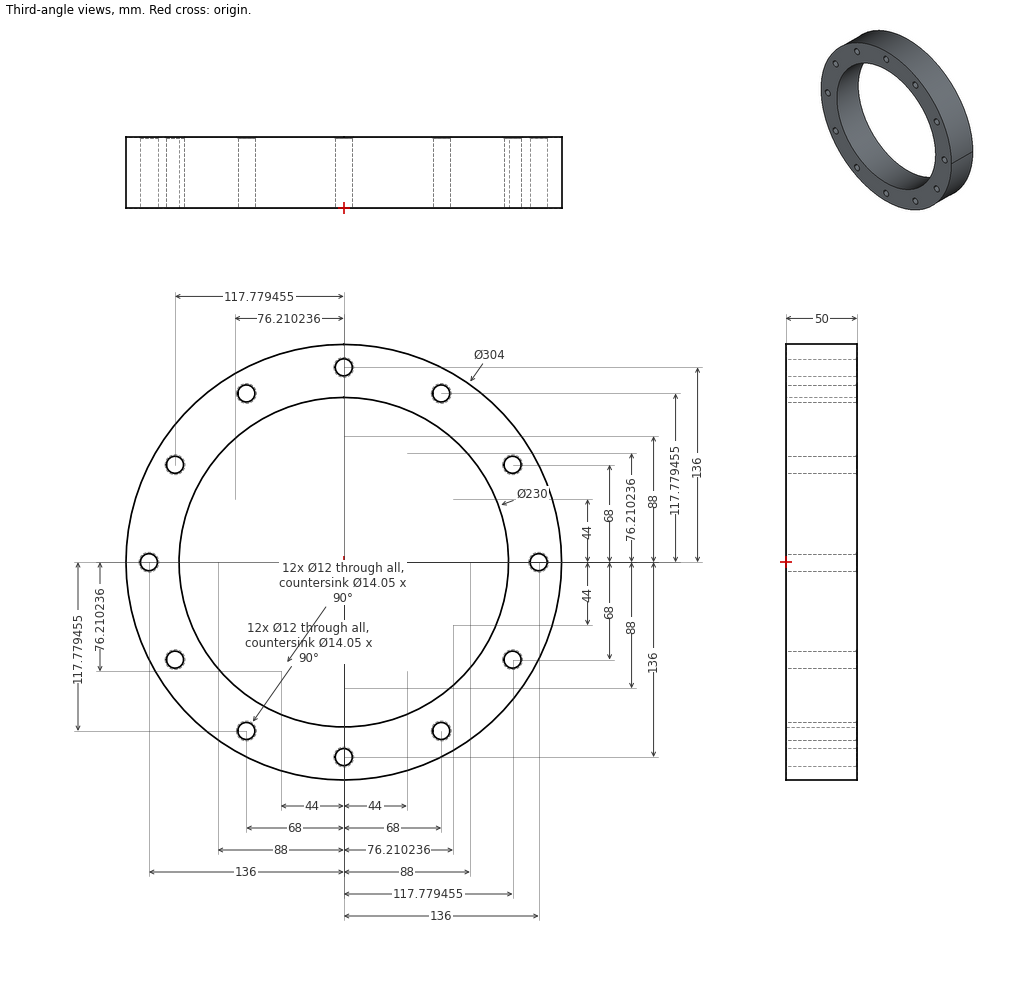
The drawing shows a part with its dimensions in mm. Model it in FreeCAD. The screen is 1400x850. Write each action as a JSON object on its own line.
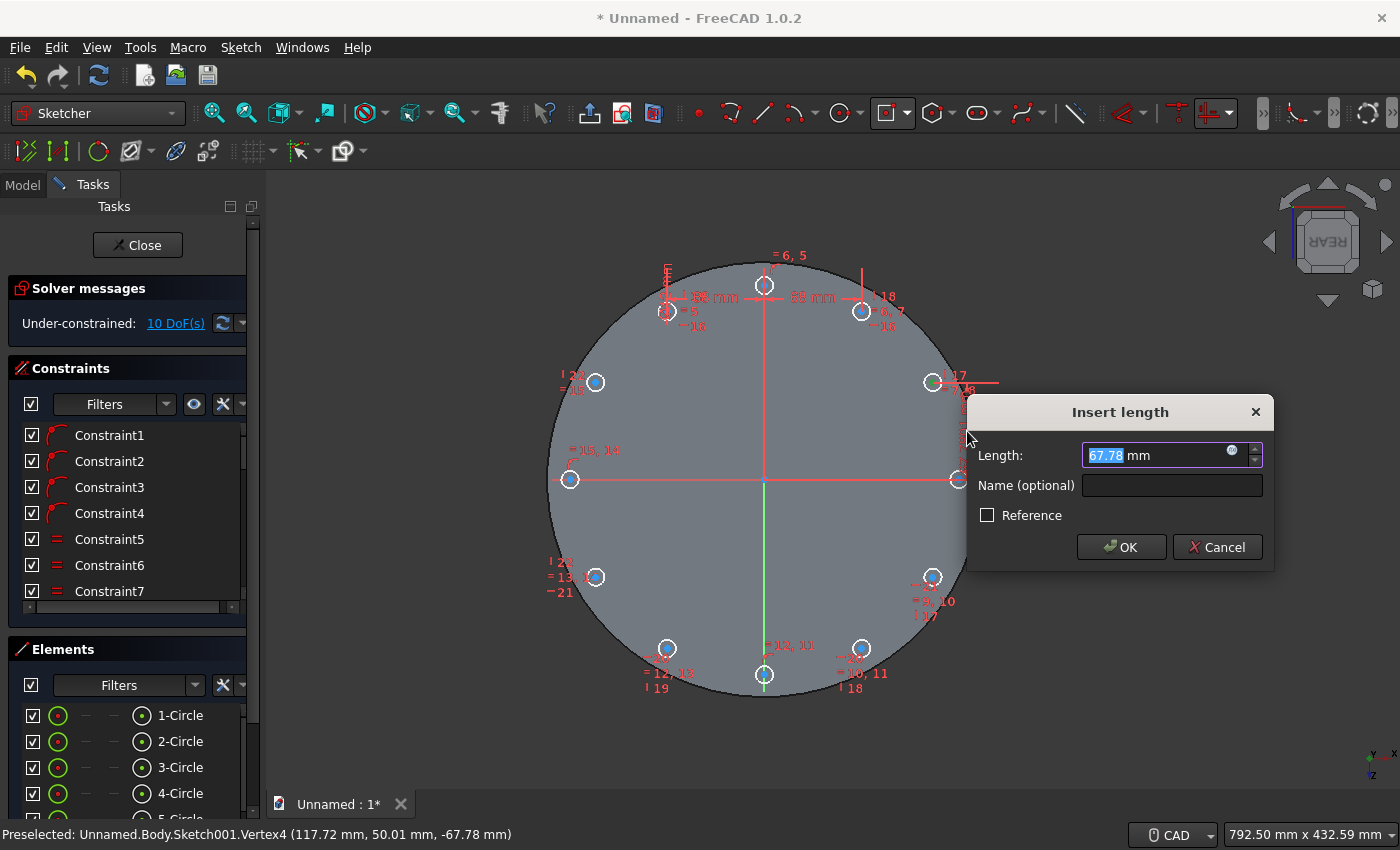
{"action": "type", "text": "68"}
{"action": "key", "text": "Return"}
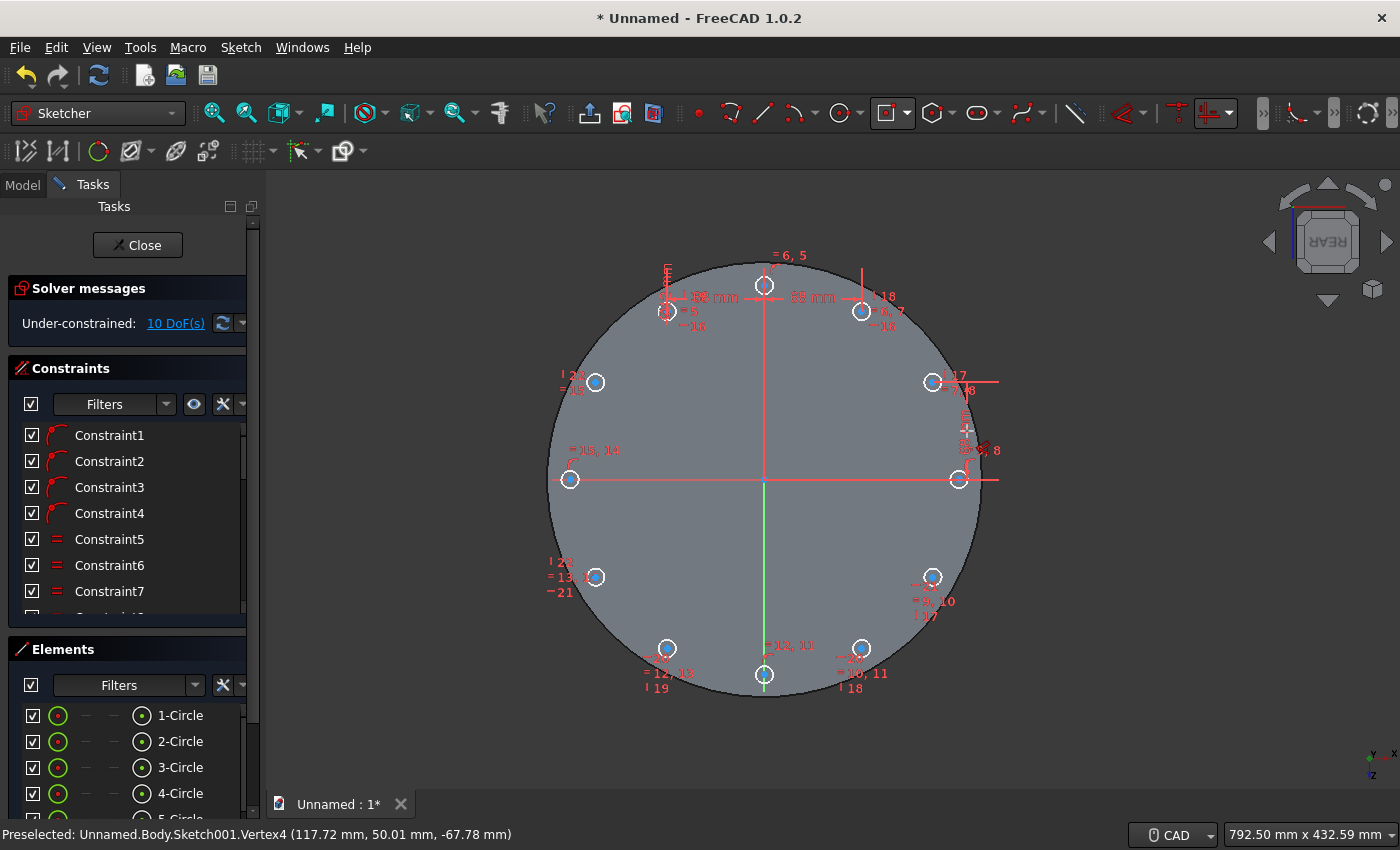
{"action": "left_click", "coordinate": [933, 577]}
{"action": "left_click", "coordinate": [967, 528]}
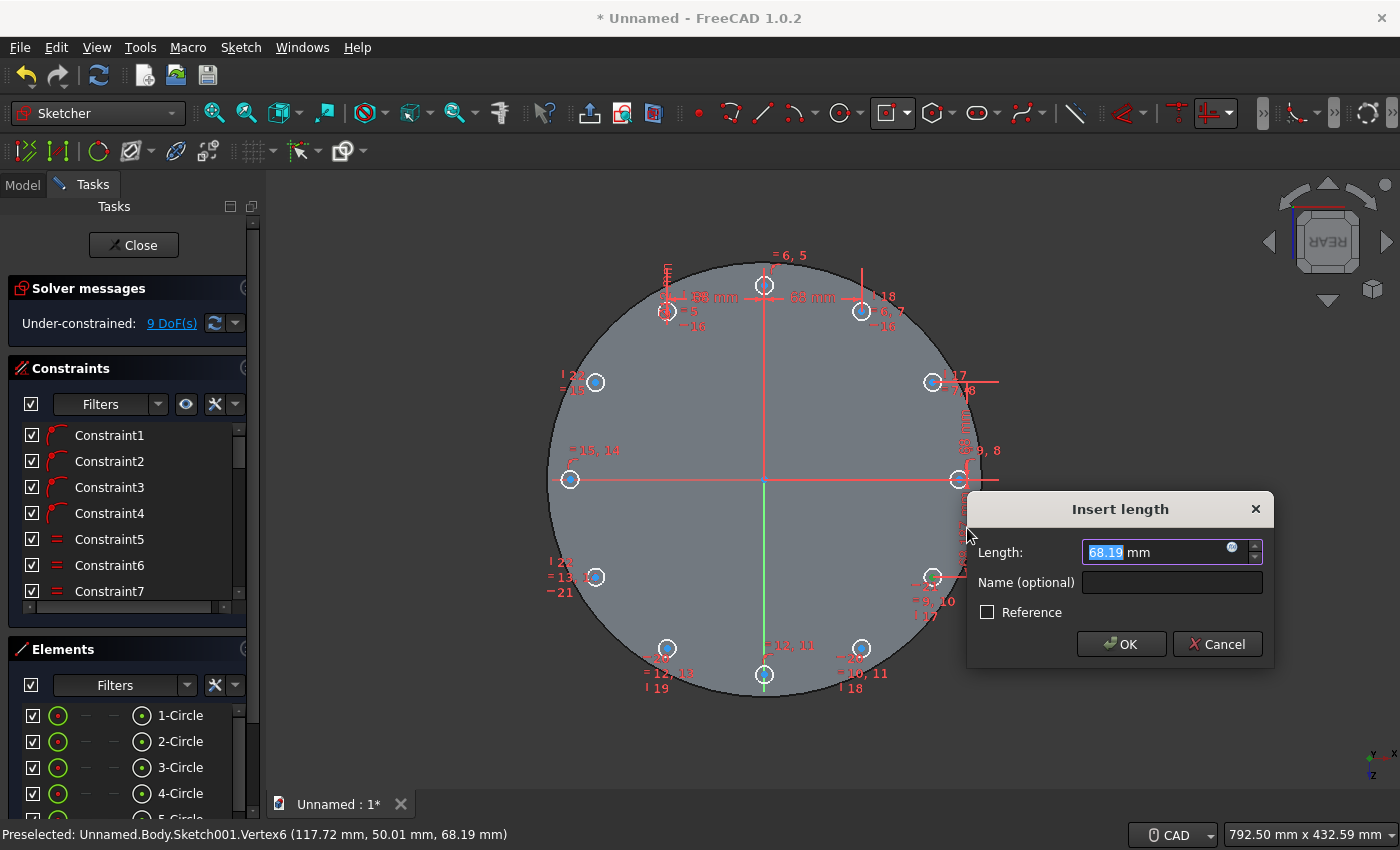
{"action": "type", "text": "68"}
{"action": "key", "text": "Return"}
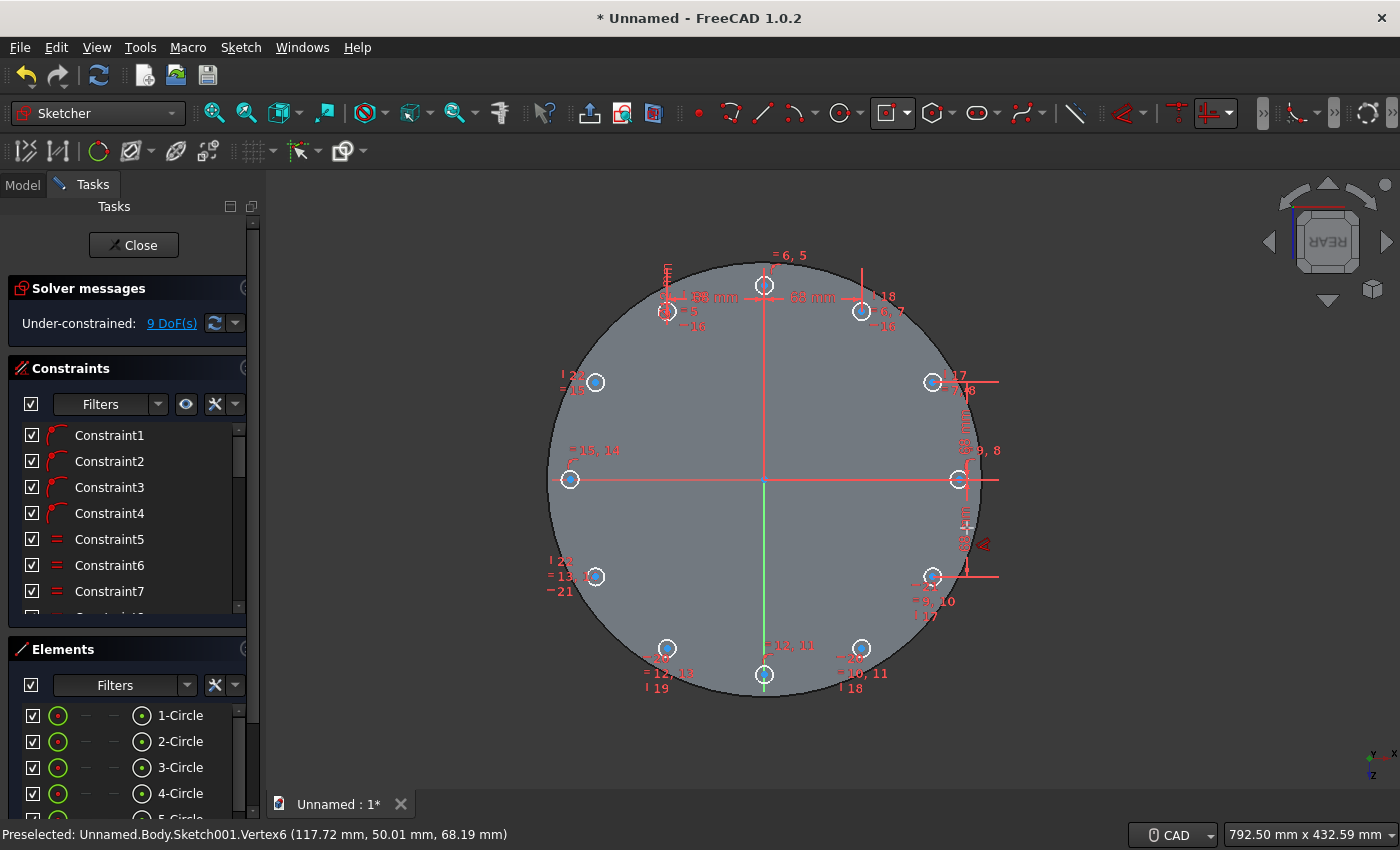
{"action": "left_click", "coordinate": [596, 383]}
{"action": "left_click", "coordinate": [562, 431]}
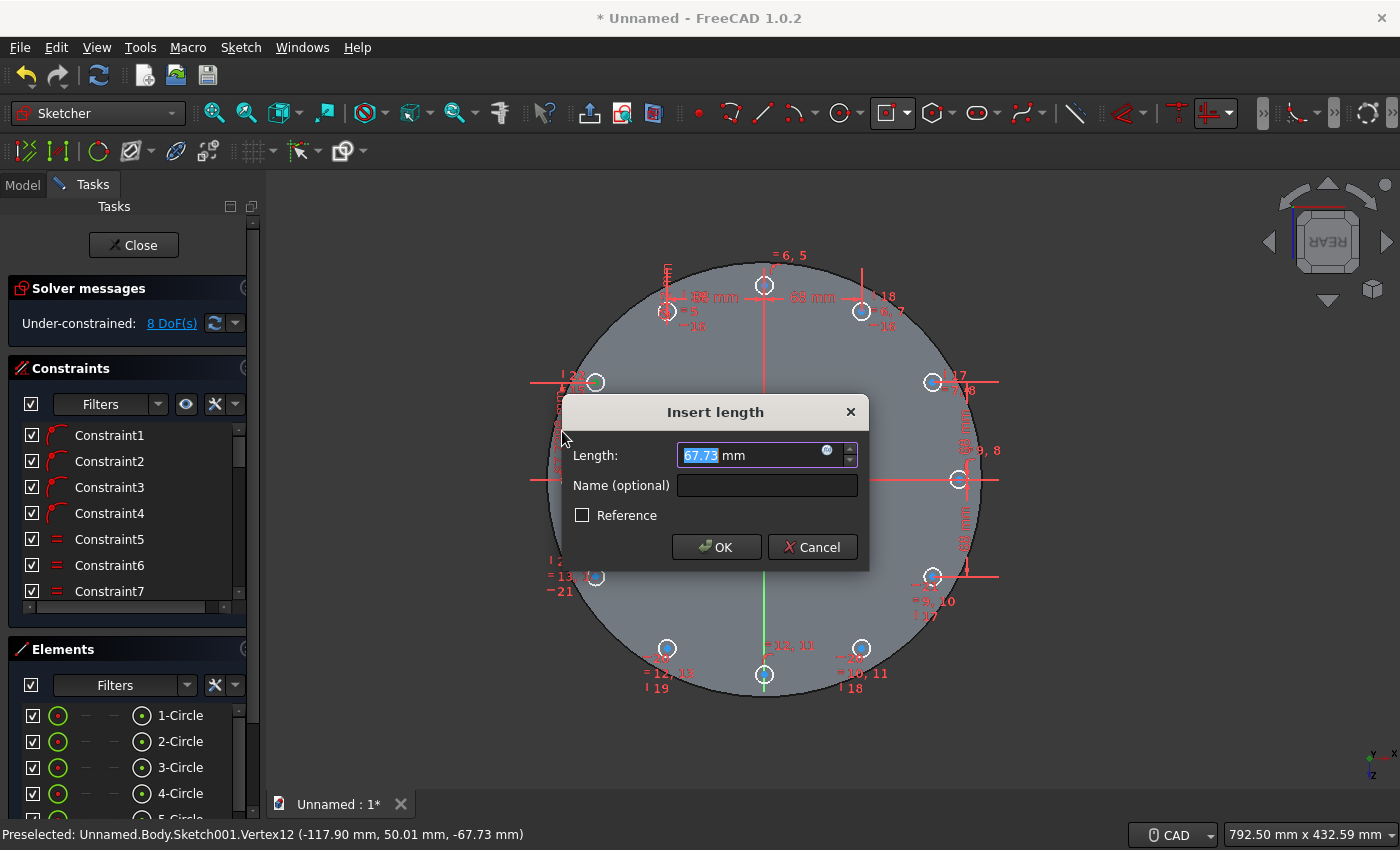
{"action": "type", "text": "68"}
{"action": "key", "text": "Return"}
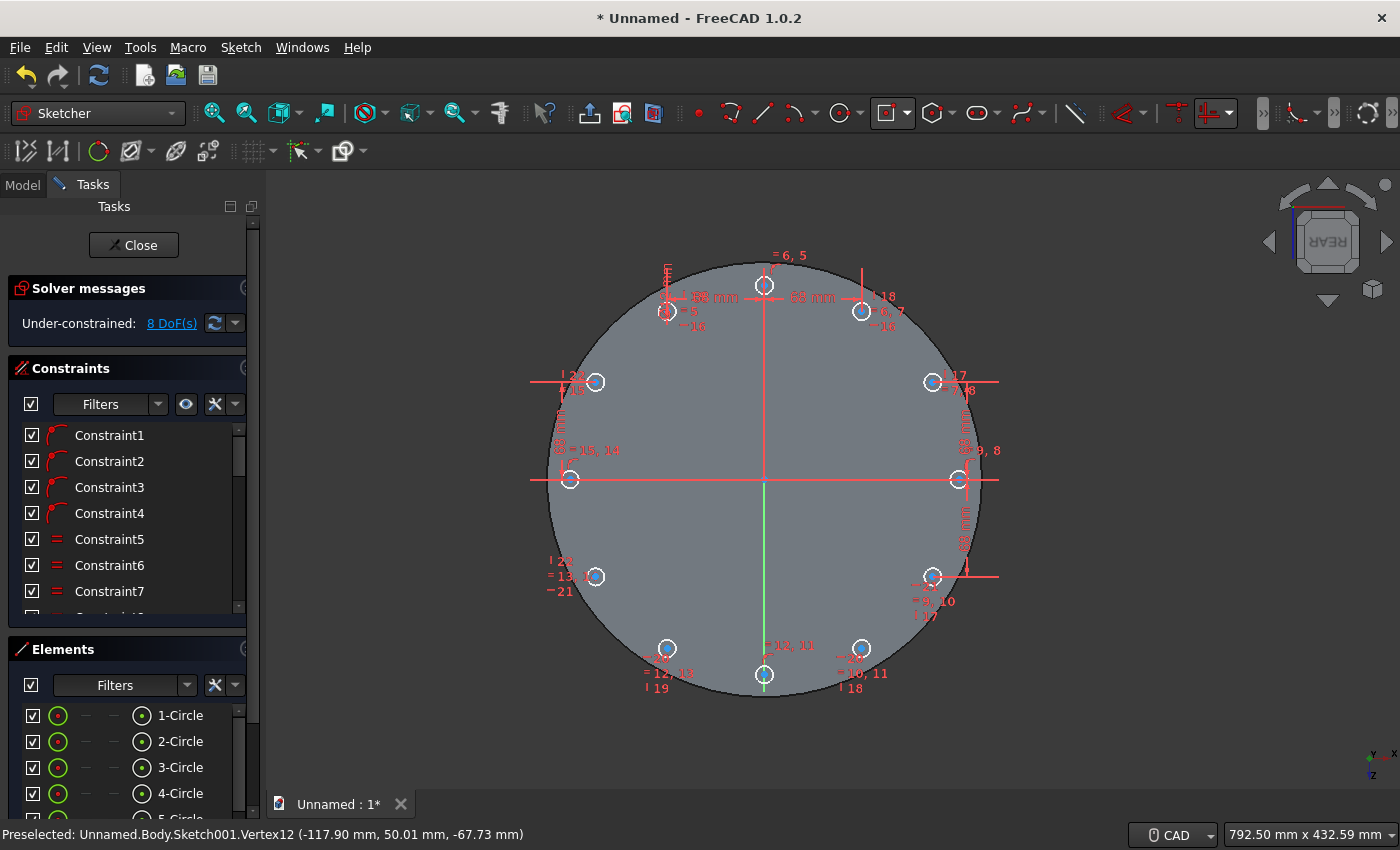
{"action": "left_click", "coordinate": [765, 286]}
{"action": "left_click", "coordinate": [799, 383]}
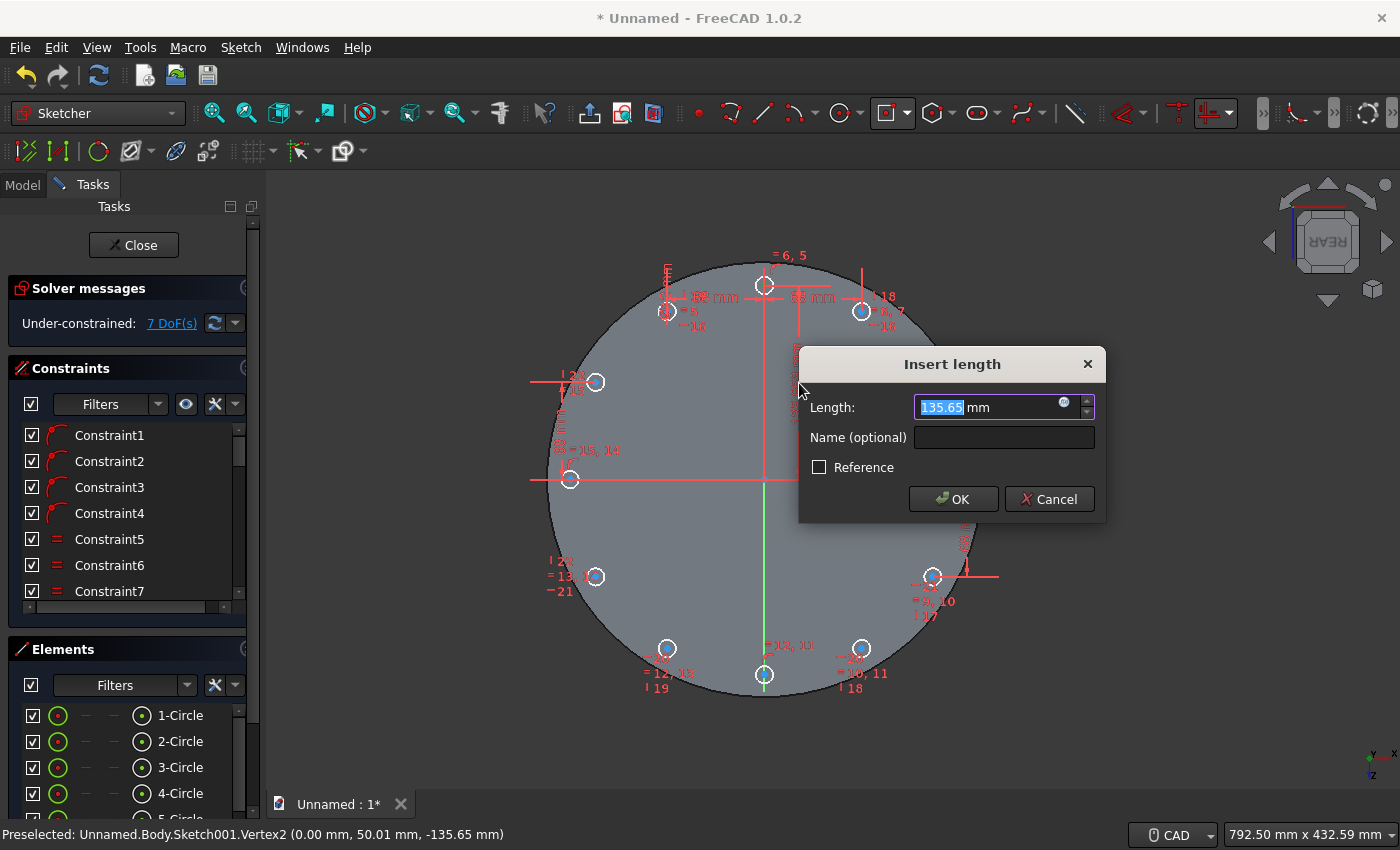
{"action": "type", "text": "136"}
{"action": "key", "text": "Return"}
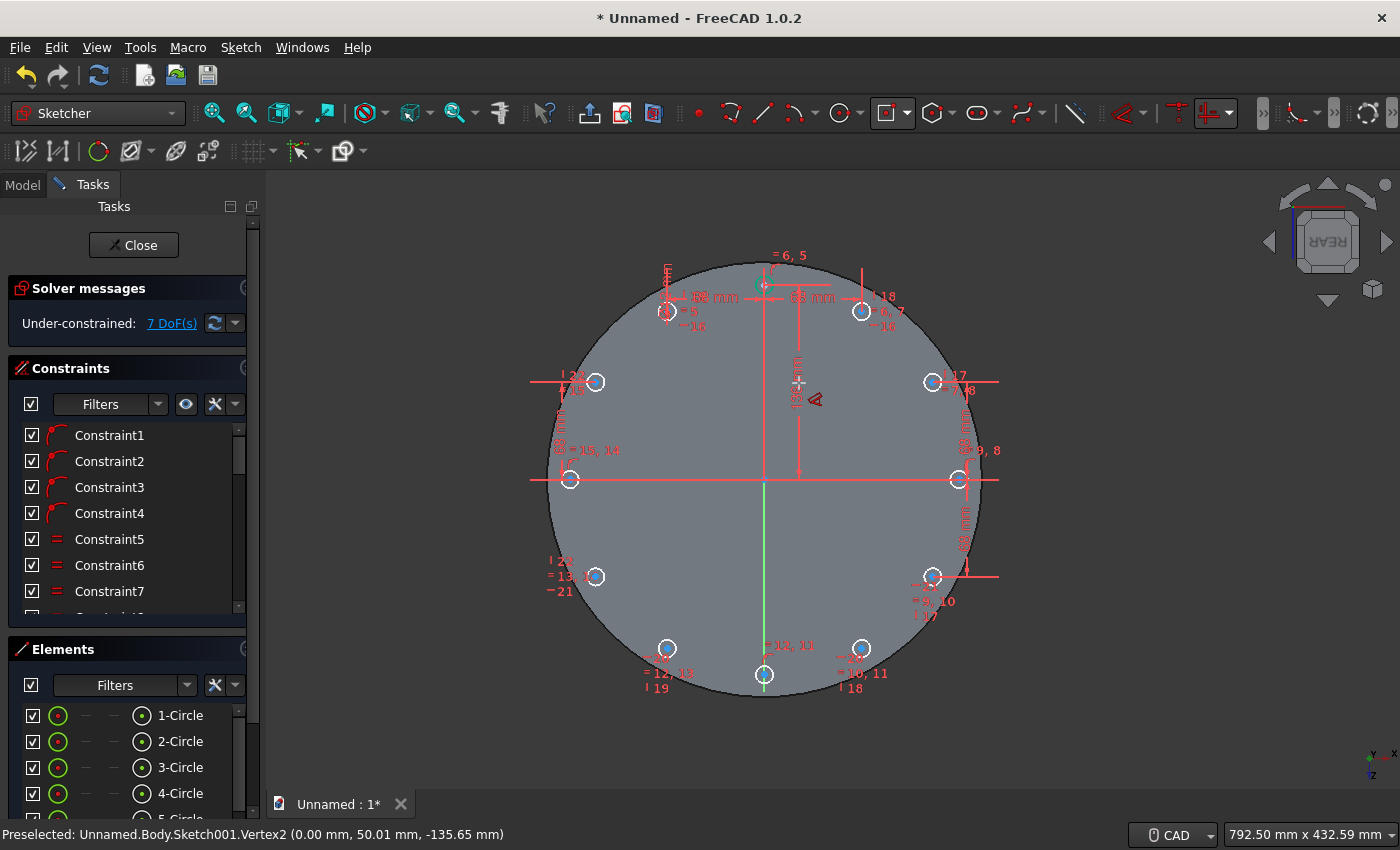
{"action": "left_click", "coordinate": [959, 480]}
{"action": "left_click", "coordinate": [862, 514]}